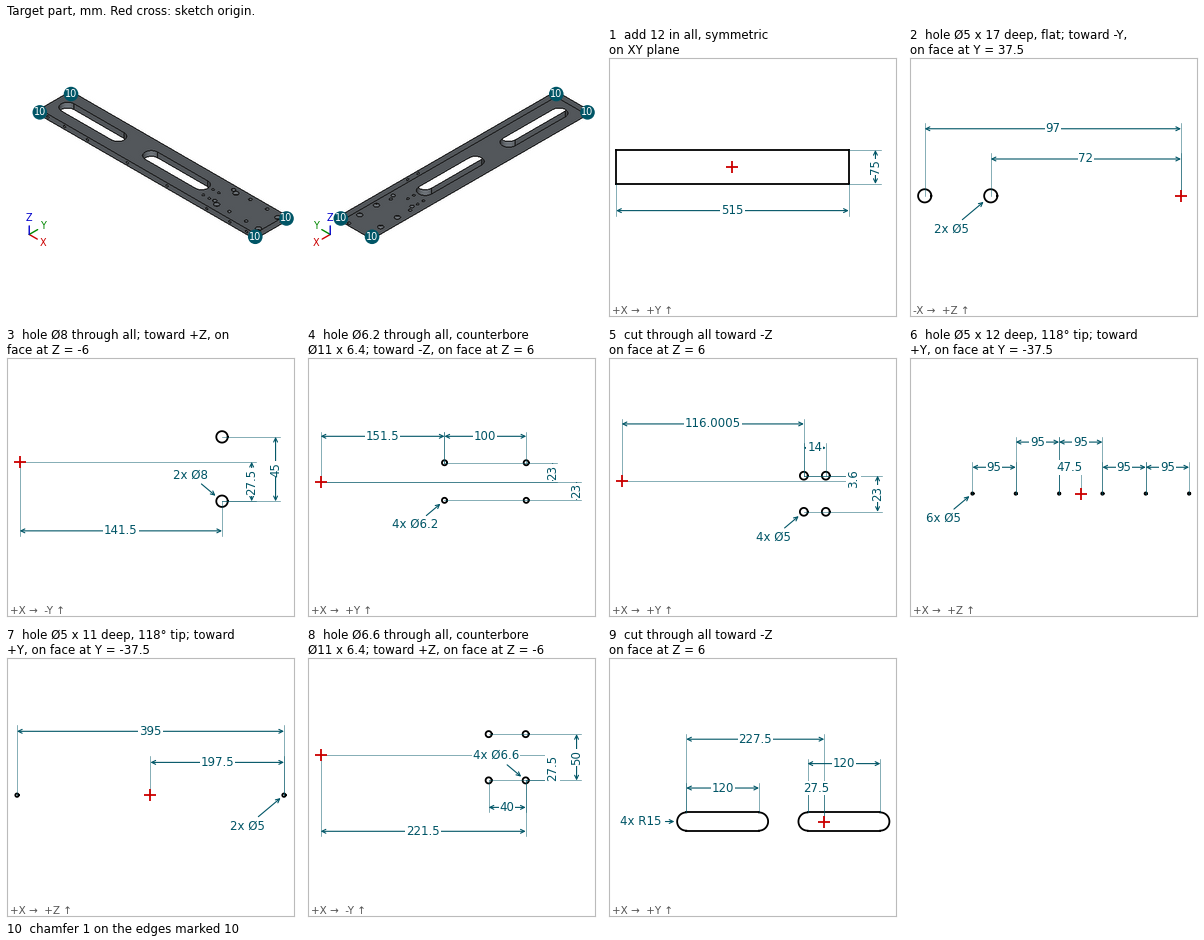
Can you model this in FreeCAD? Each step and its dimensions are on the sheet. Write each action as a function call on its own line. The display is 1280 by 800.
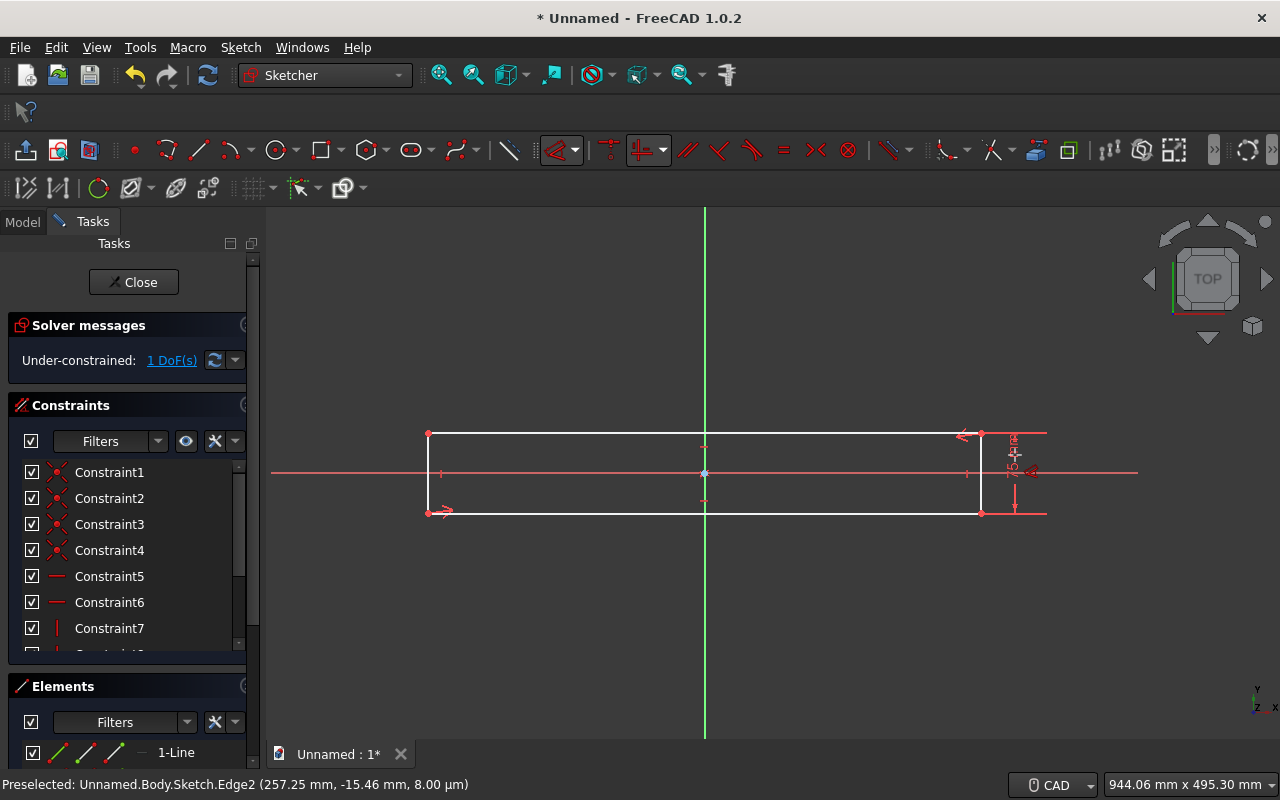
click(594, 514)
click(578, 548)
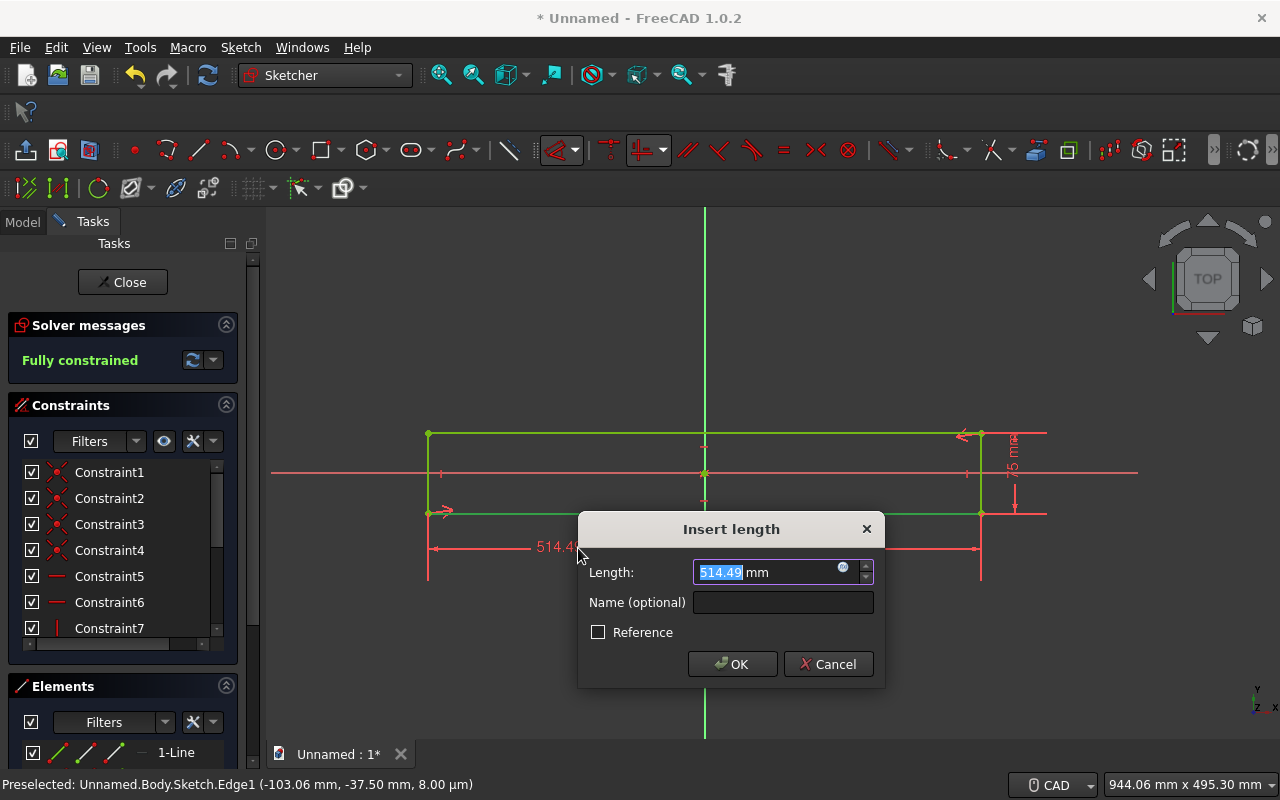
text(515)
key(Return)
key(Escape)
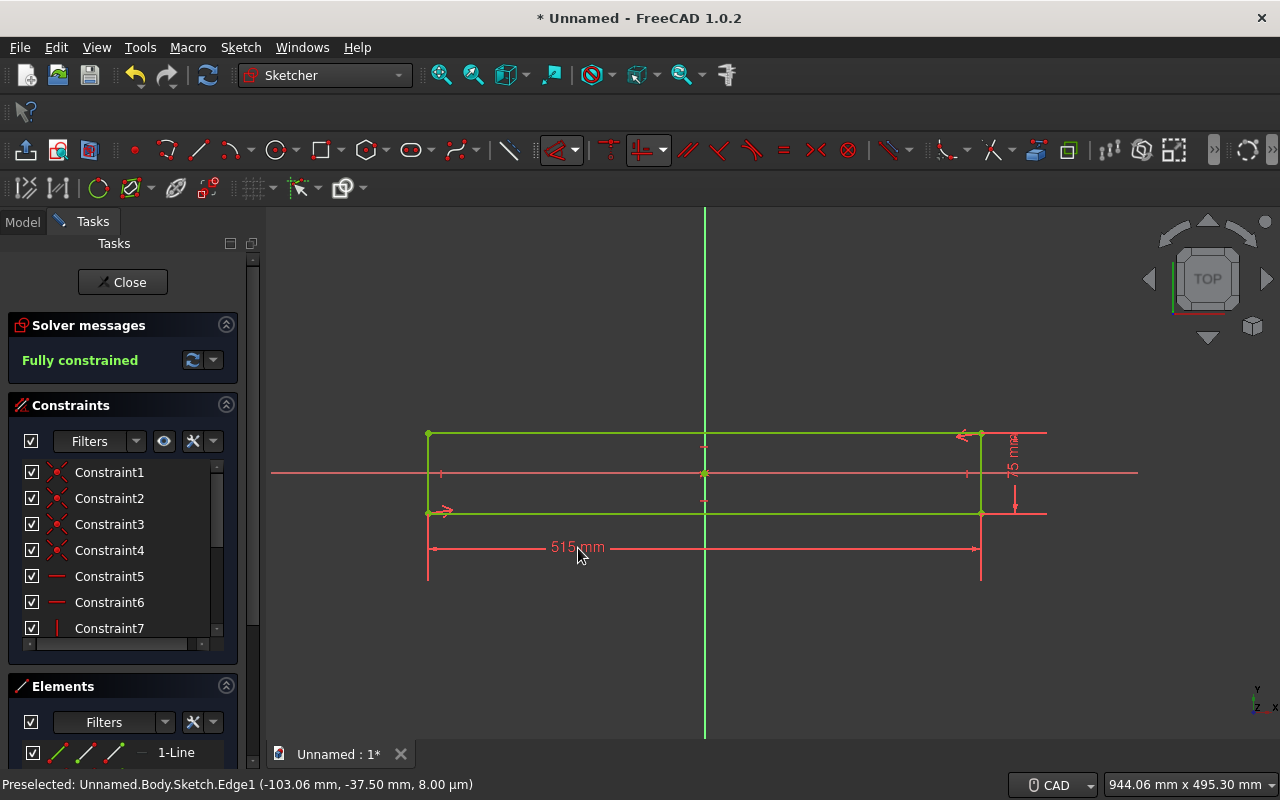
click(123, 282)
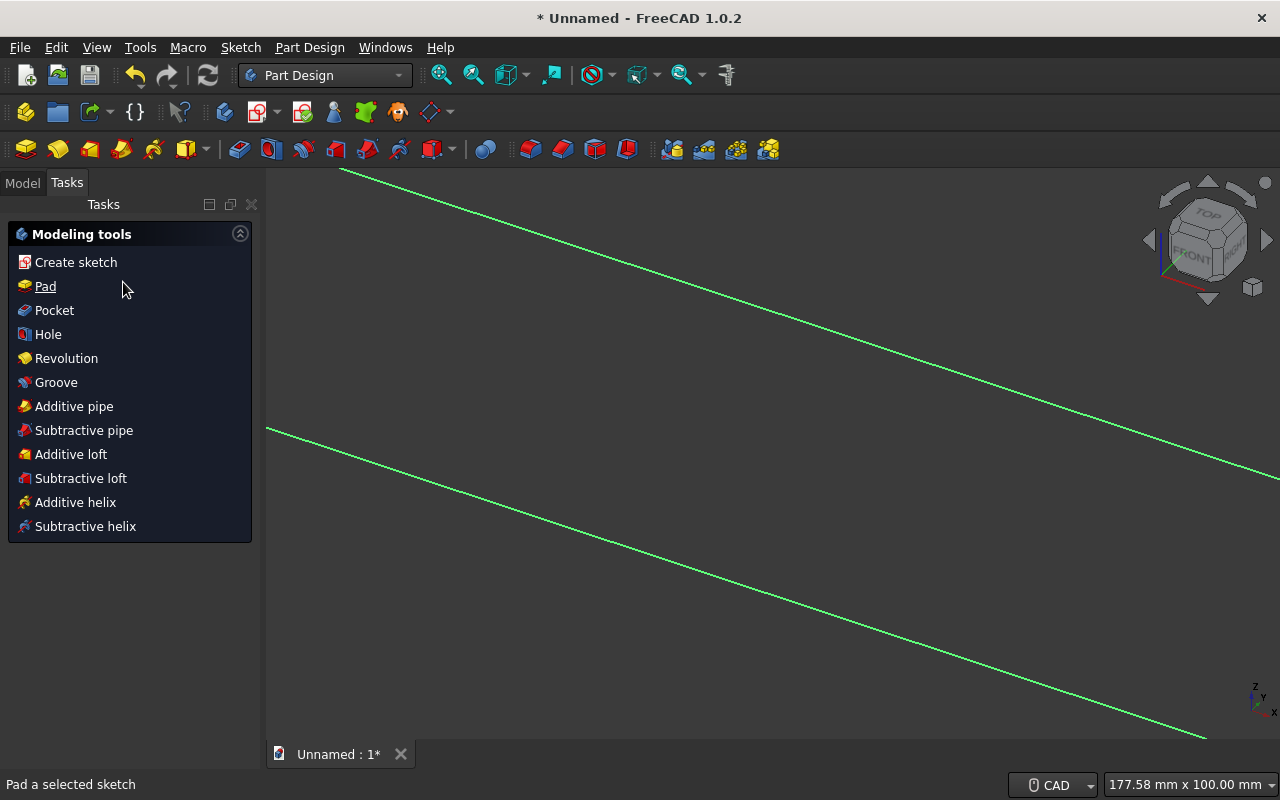
click(26, 150)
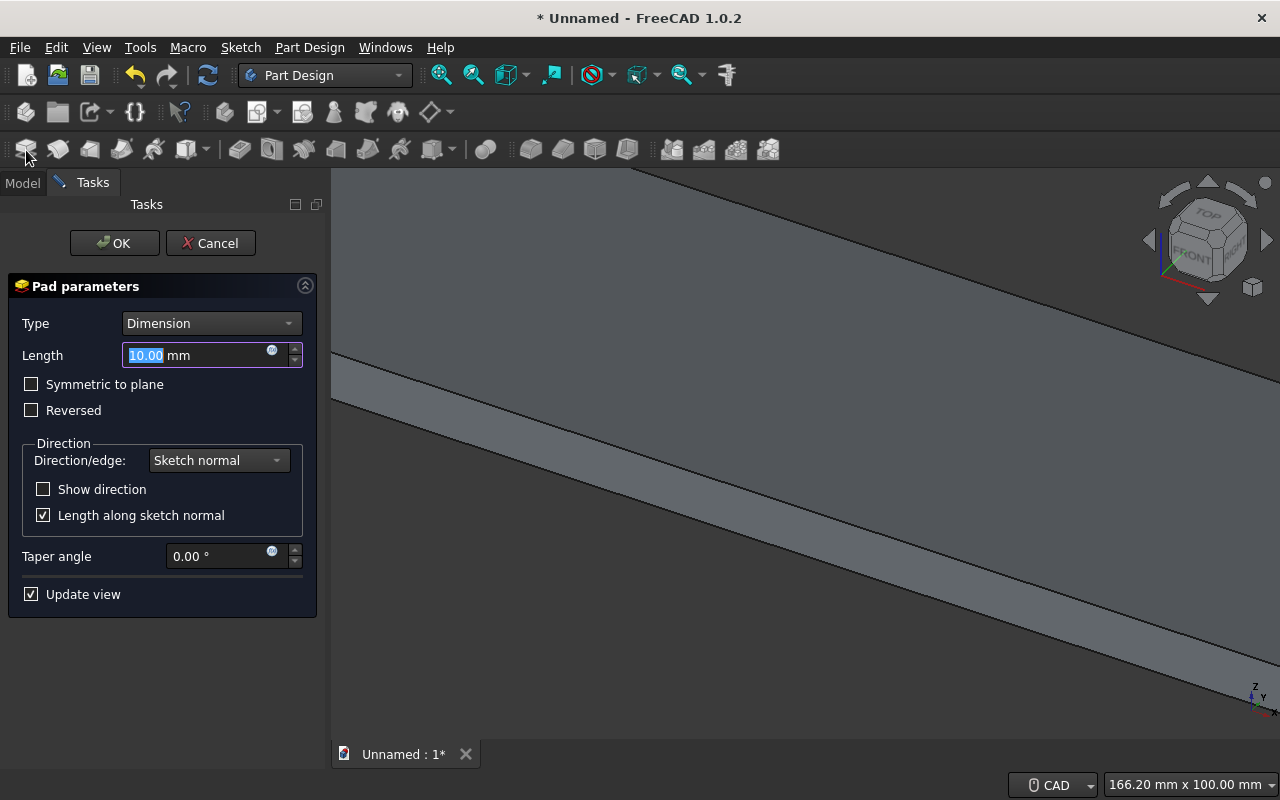
text(12)
key(Tab)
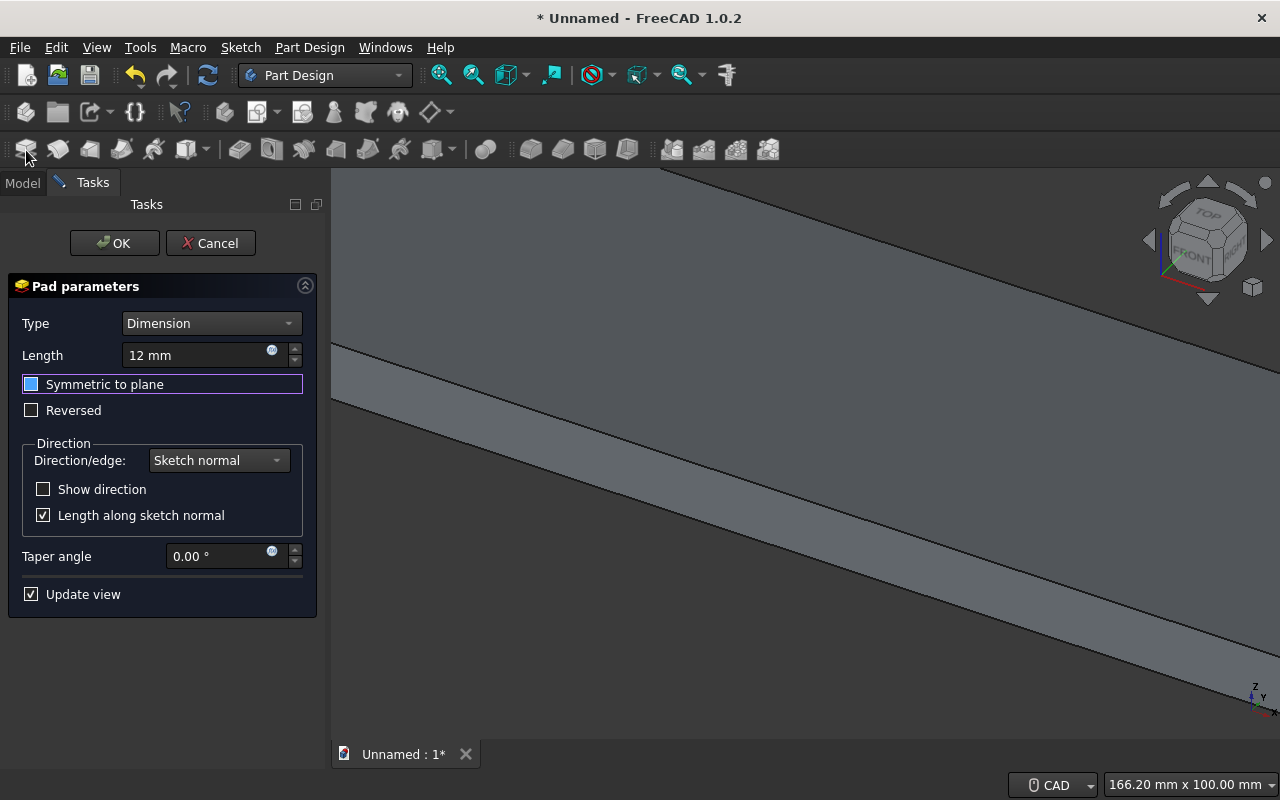
click(30, 384)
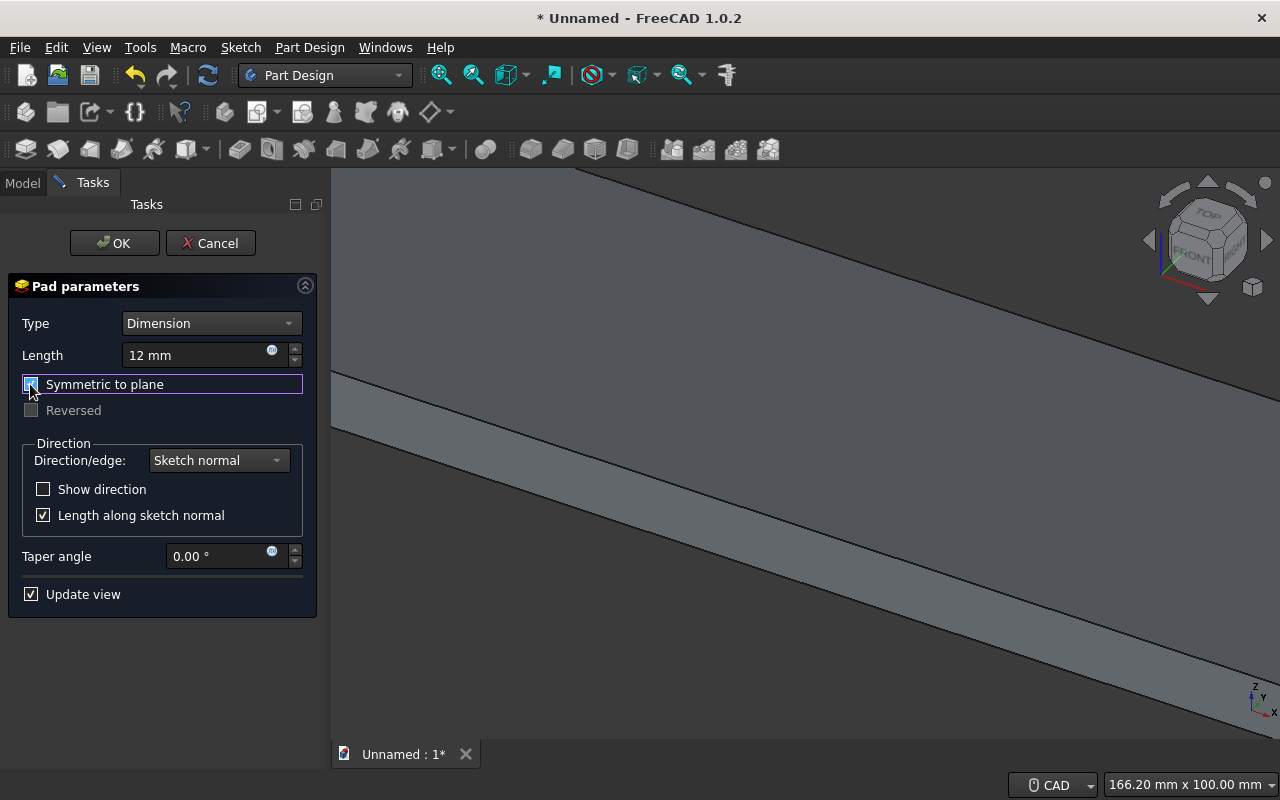
click(115, 243)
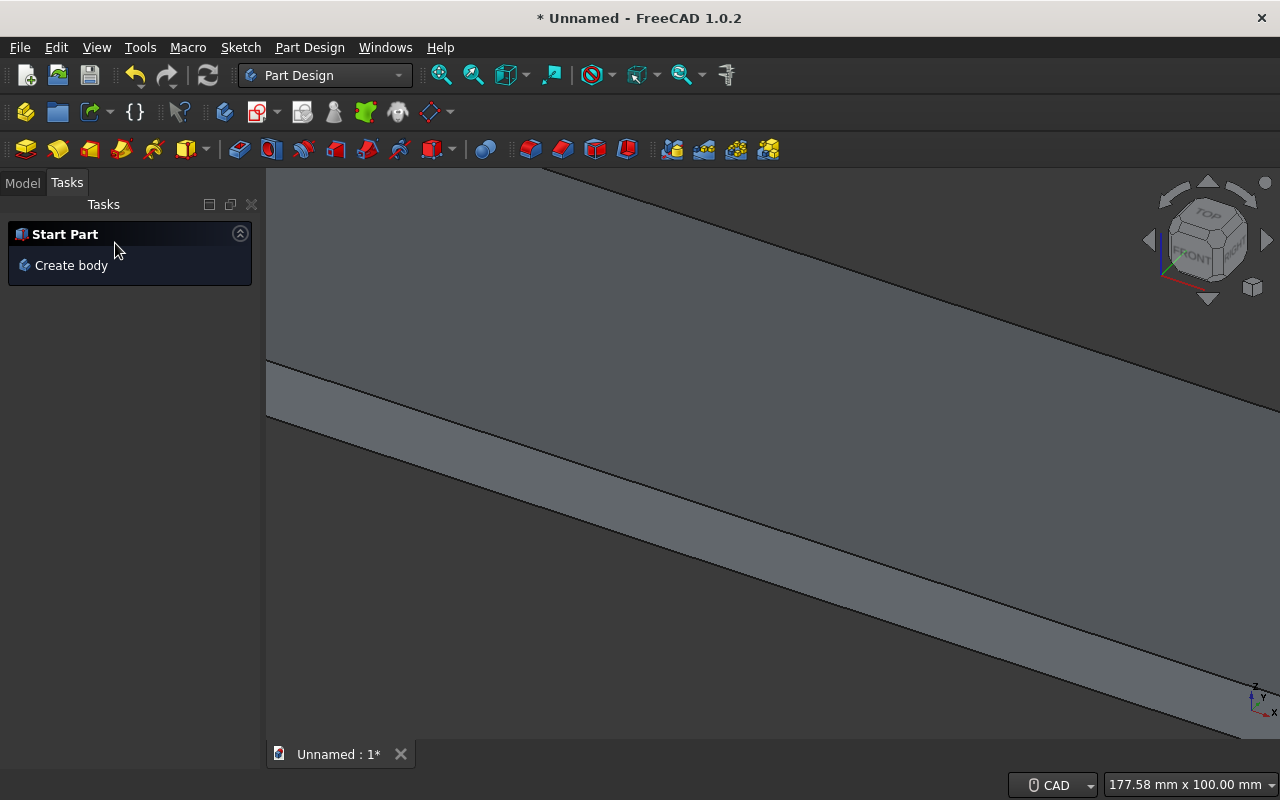
key(v)
key(f)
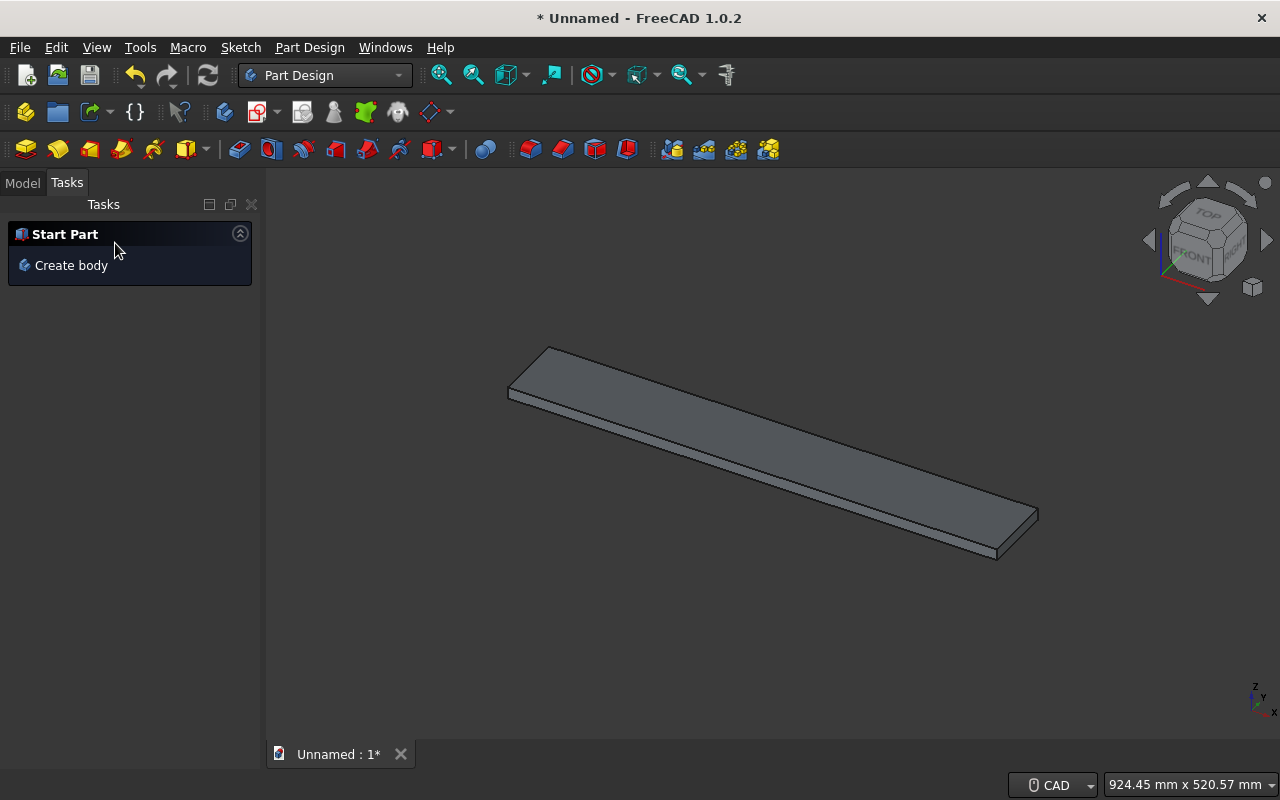
key(4)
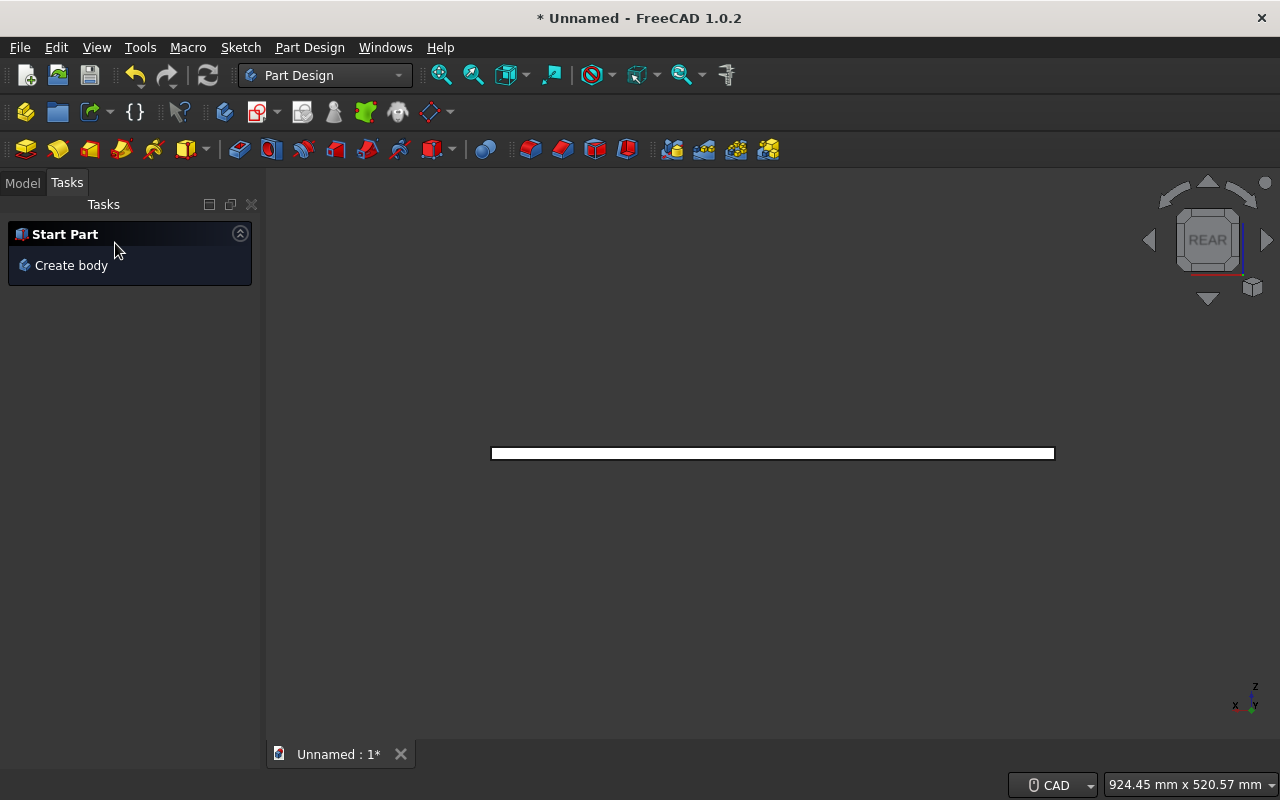
scroll(531, 452, up, 4)